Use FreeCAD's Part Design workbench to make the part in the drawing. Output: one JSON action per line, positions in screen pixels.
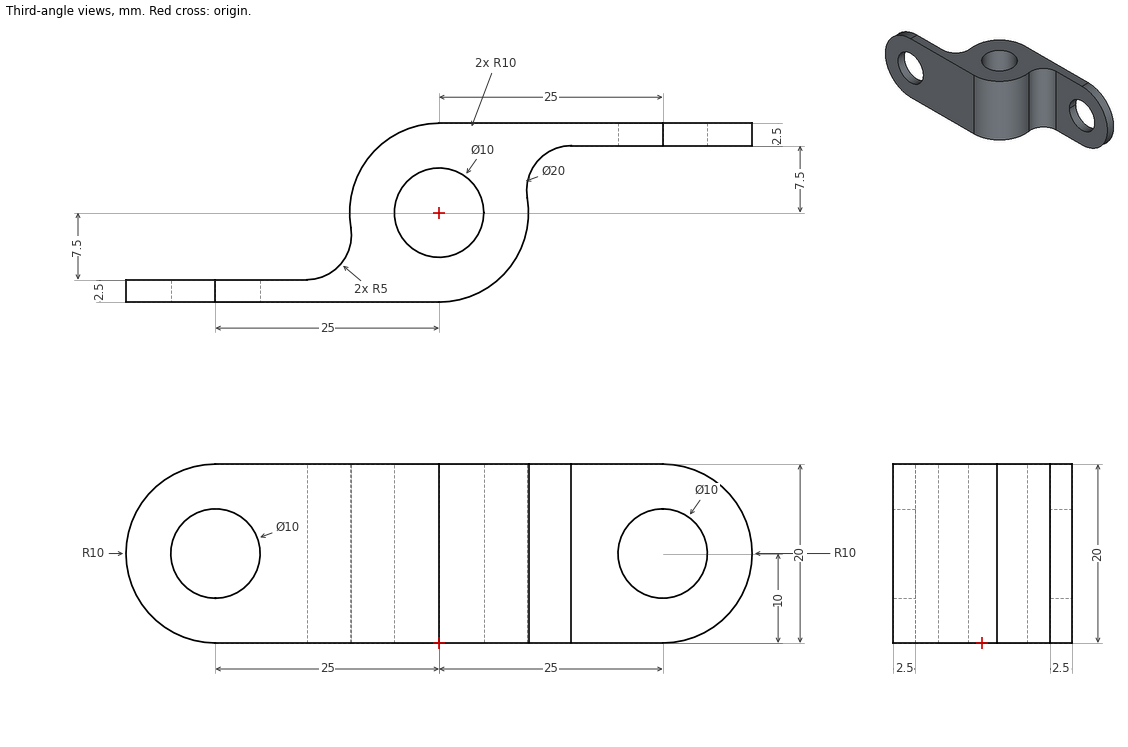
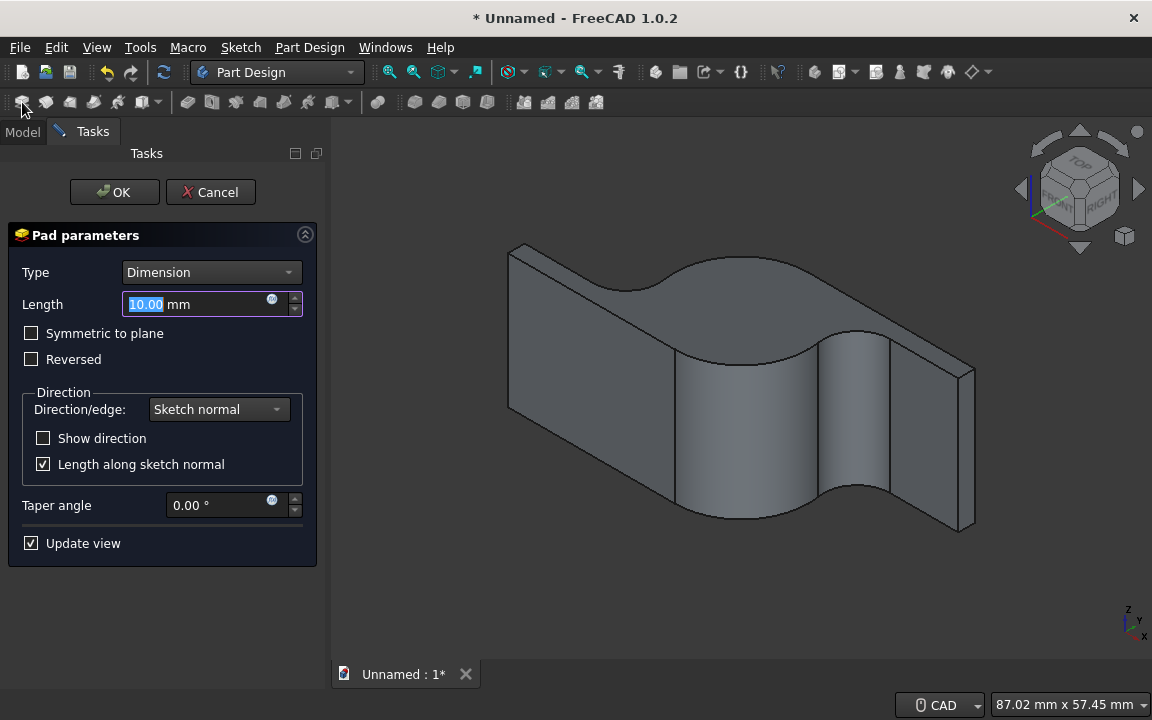
{"action": "type", "text": "2.5"}
{"action": "key", "text": "Tab"}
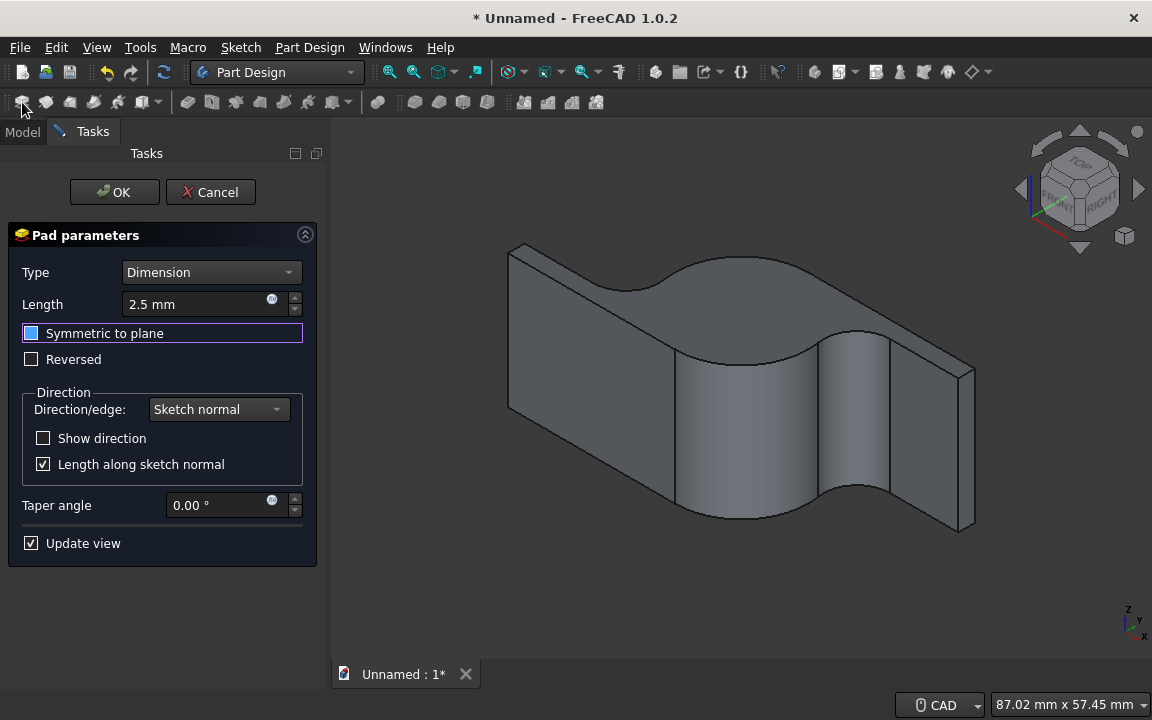
{"action": "left_click", "coordinate": [30, 359]}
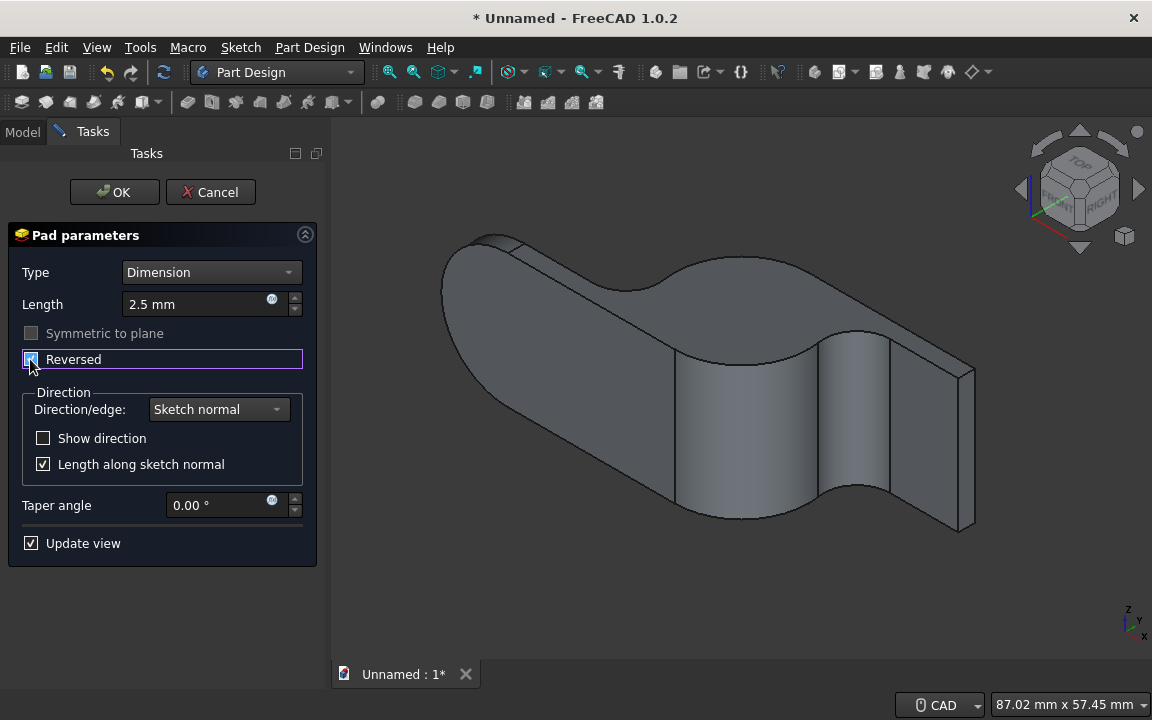
{"action": "left_click", "coordinate": [115, 192]}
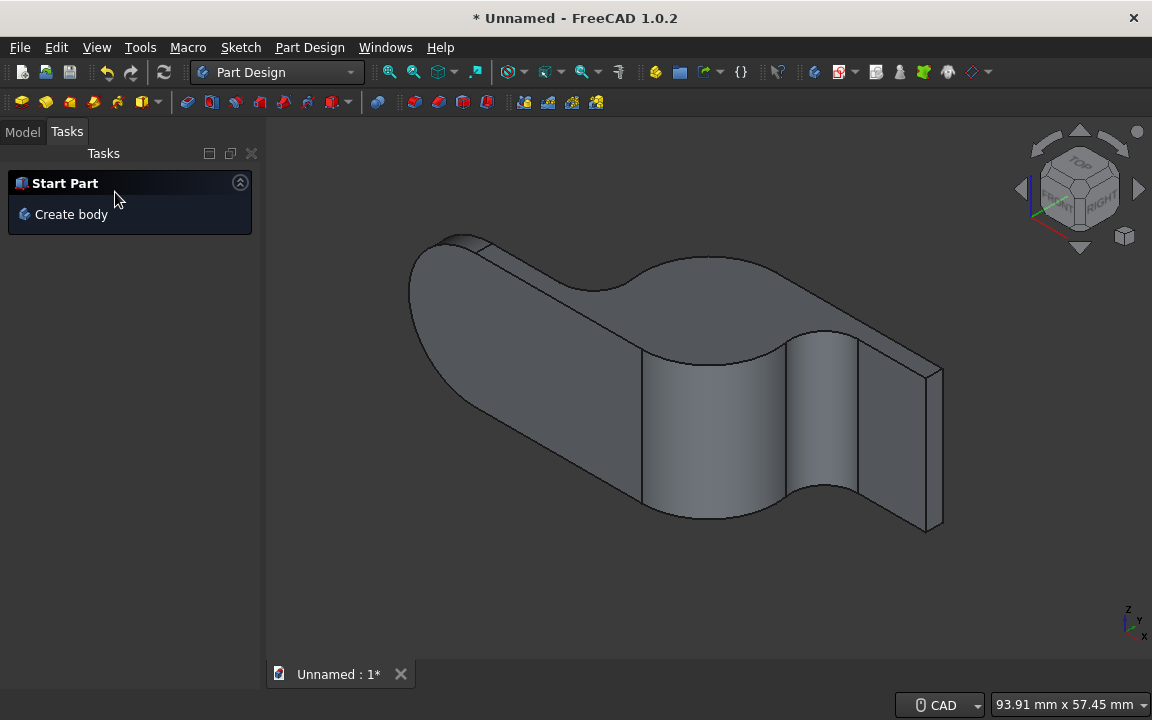
{"action": "key", "text": "4"}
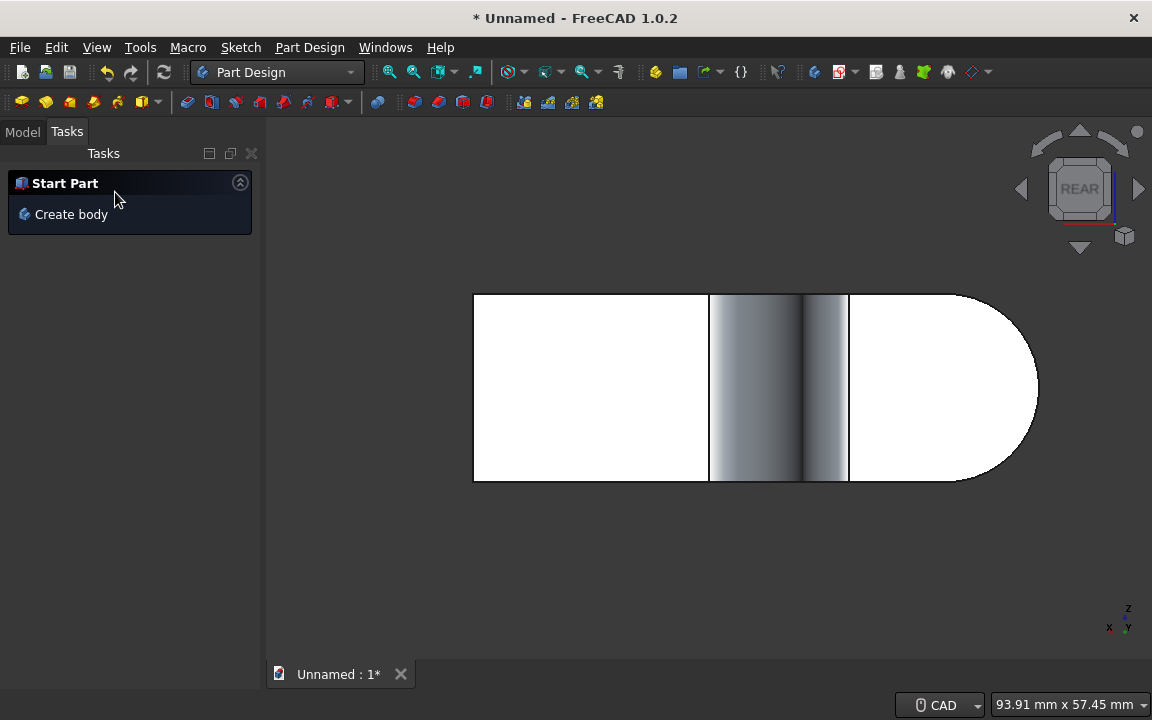
{"action": "left_click", "coordinate": [591, 387]}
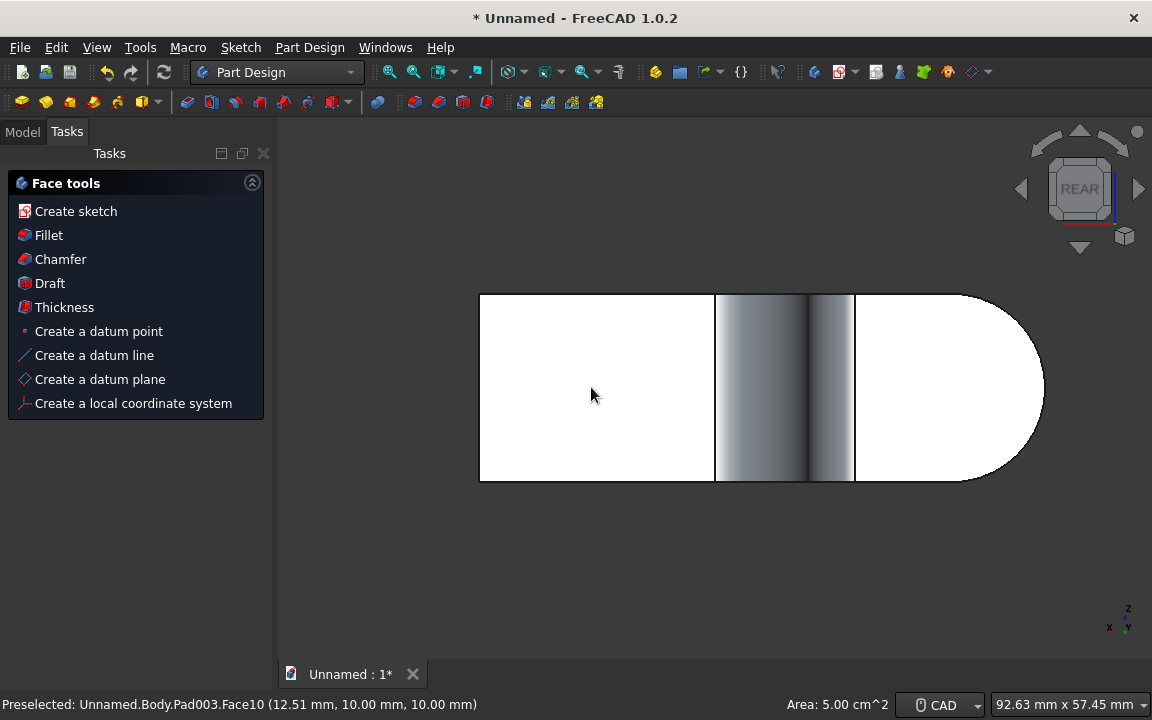
{"action": "left_click", "coordinate": [840, 72]}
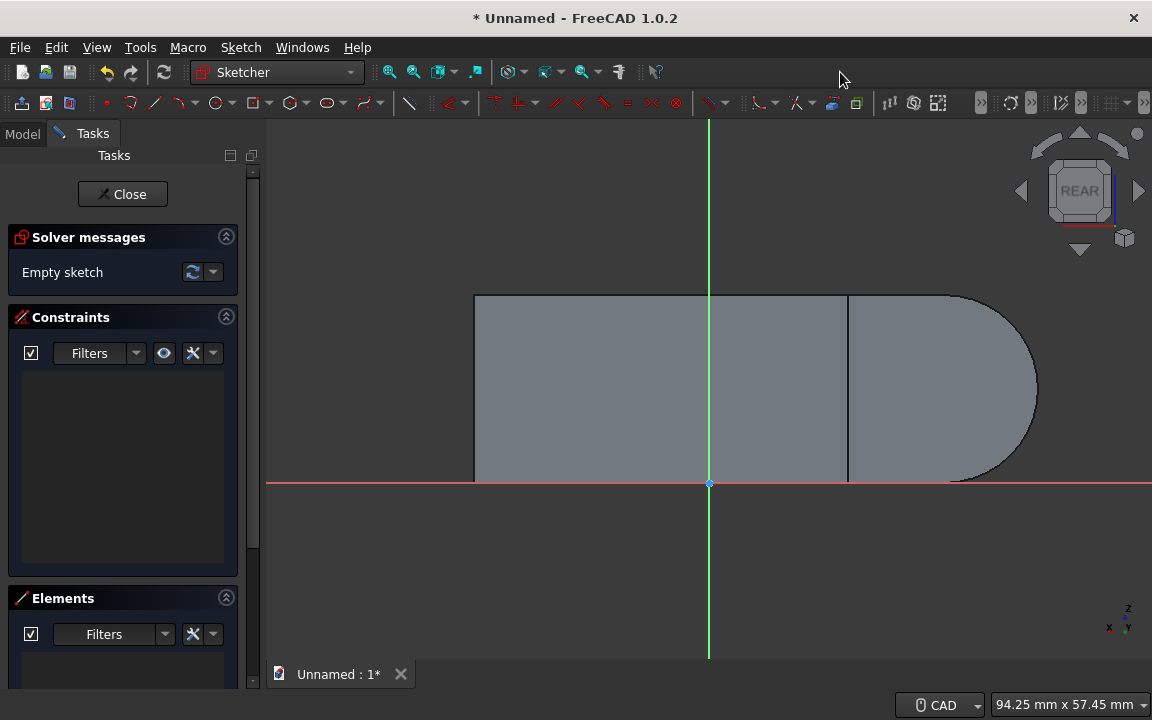
{"action": "scroll", "coordinate": [349, 389], "scroll_direction": "up", "scroll_amount": 2}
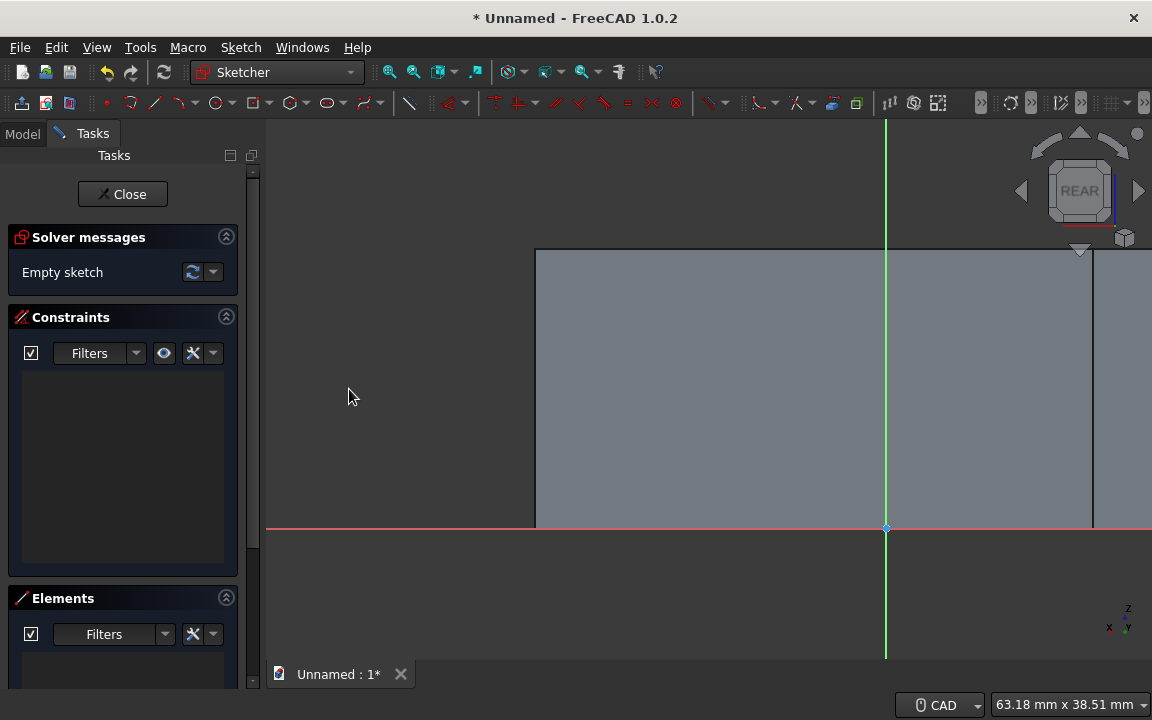
{"action": "left_click", "coordinate": [156, 104]}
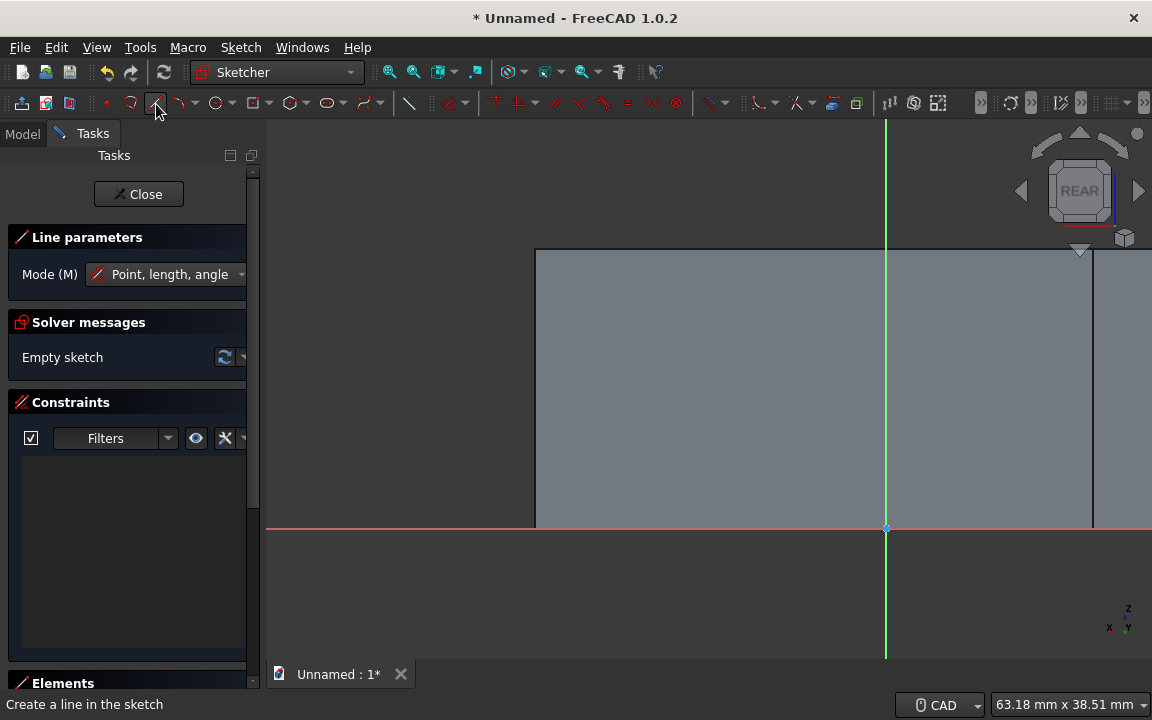
{"action": "left_click", "coordinate": [535, 529]}
{"action": "left_click", "coordinate": [535, 249]}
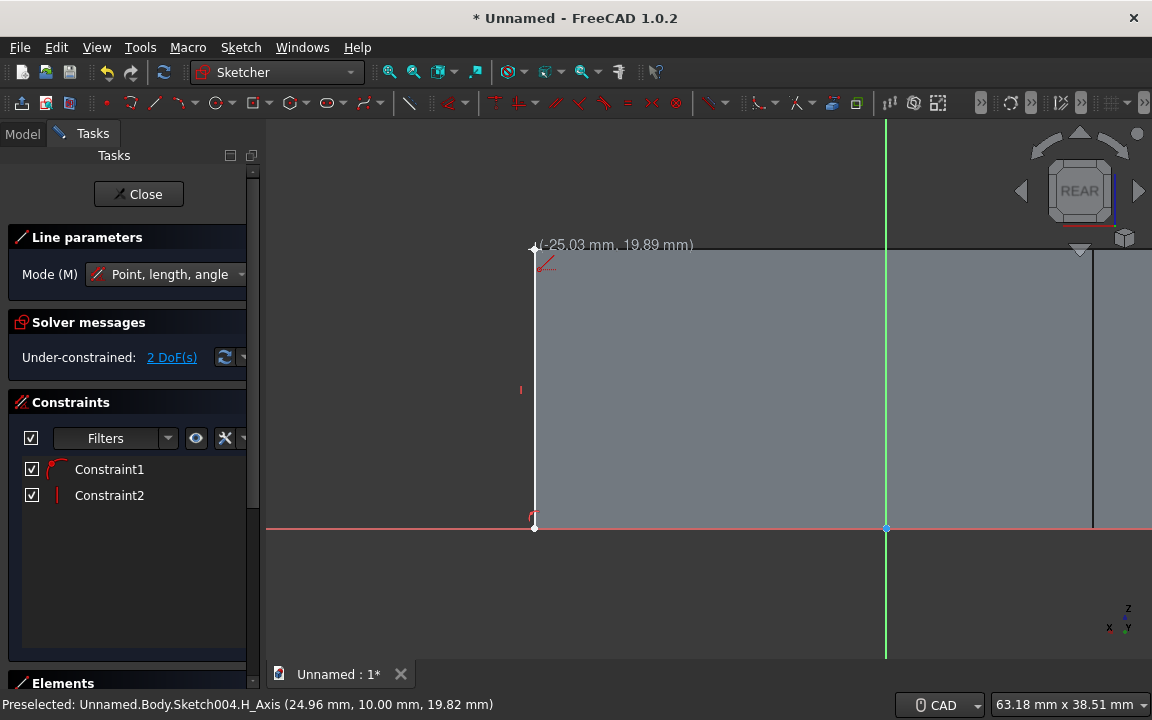
{"action": "left_click", "coordinate": [180, 104]}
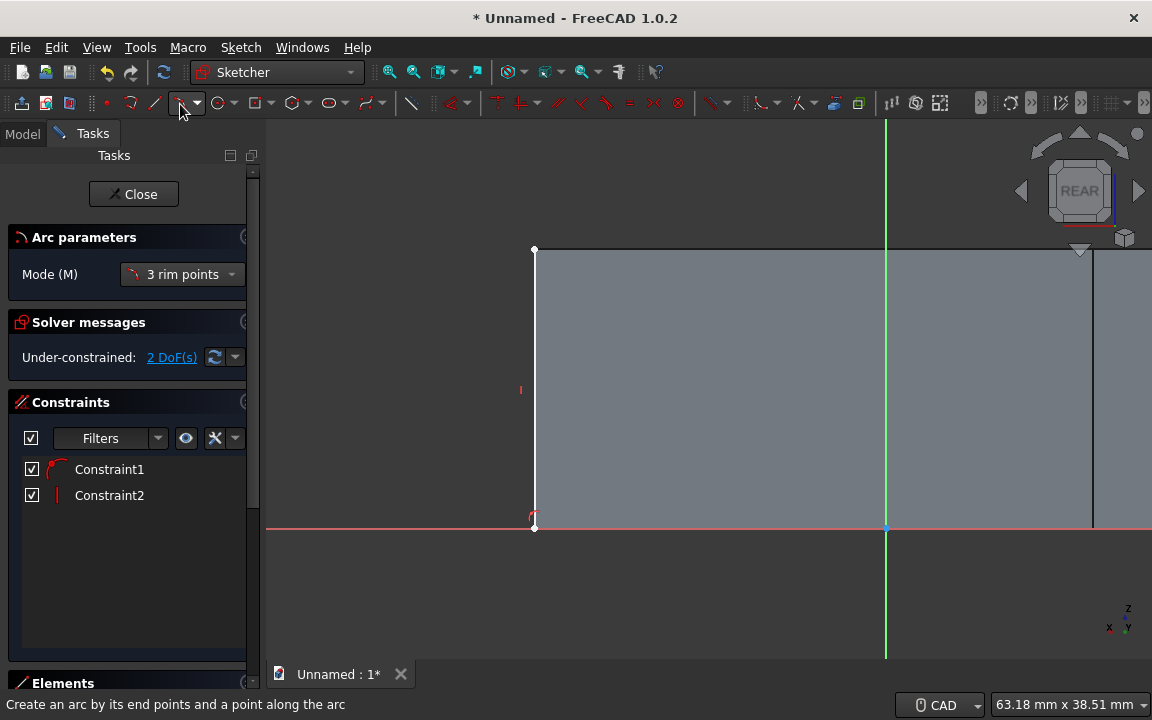
{"action": "left_click", "coordinate": [535, 250]}
{"action": "left_click", "coordinate": [535, 529]}
{"action": "left_click", "coordinate": [395, 389]}
{"action": "key", "text": "Escape"}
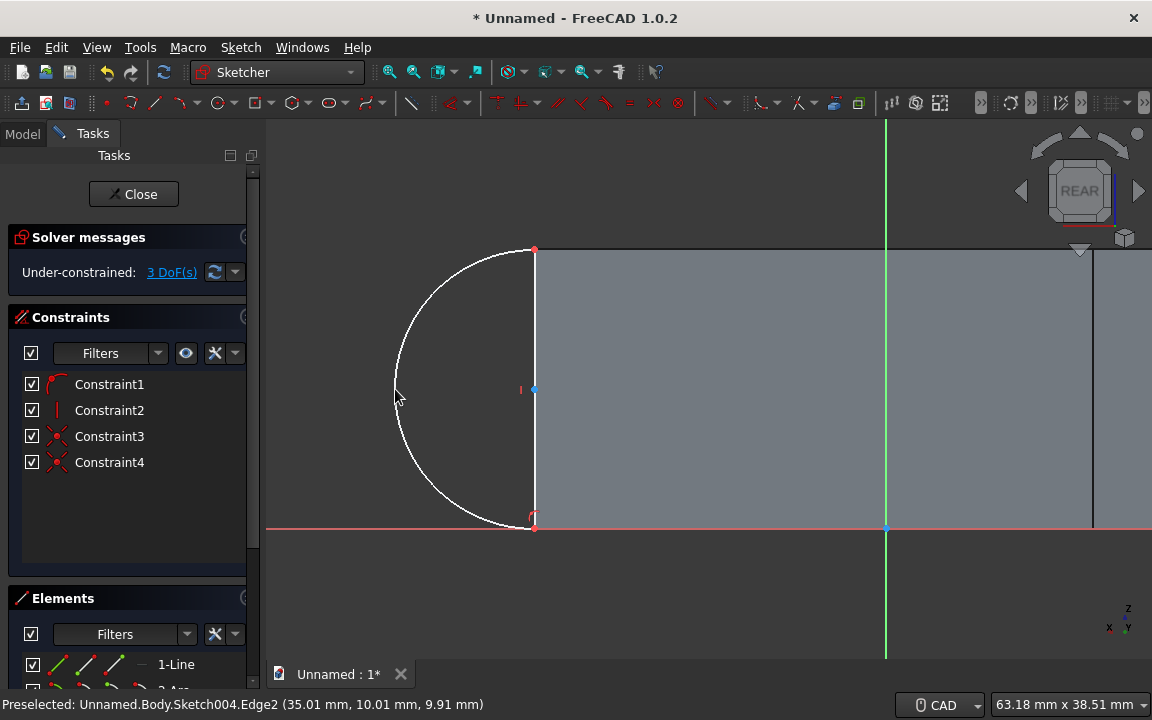
{"action": "key", "text": "d"}